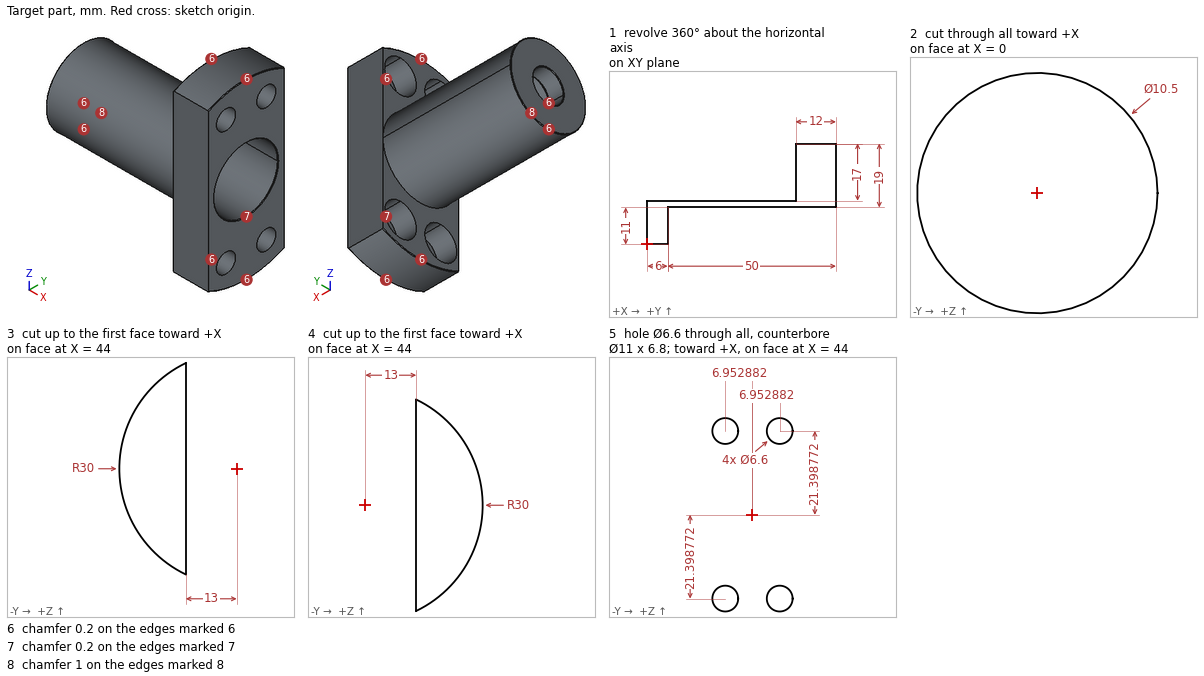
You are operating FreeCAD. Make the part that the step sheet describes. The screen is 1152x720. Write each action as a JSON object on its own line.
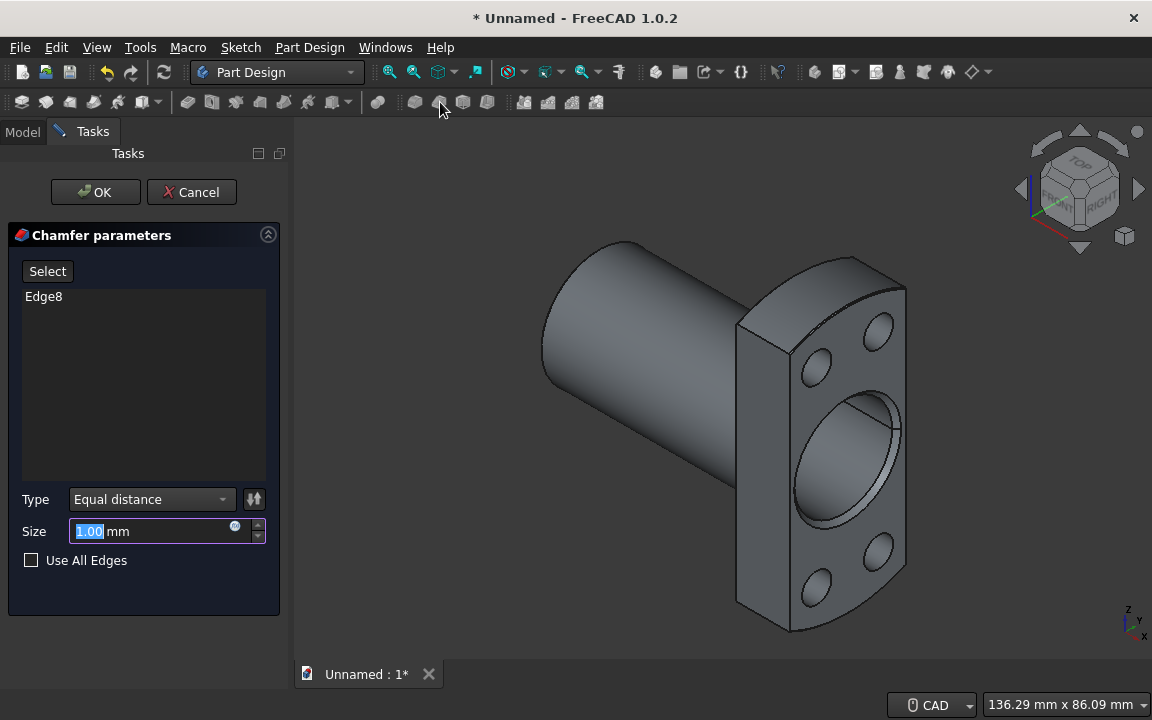
{"action": "type", "text": "0.2"}
{"action": "key", "text": "Tab"}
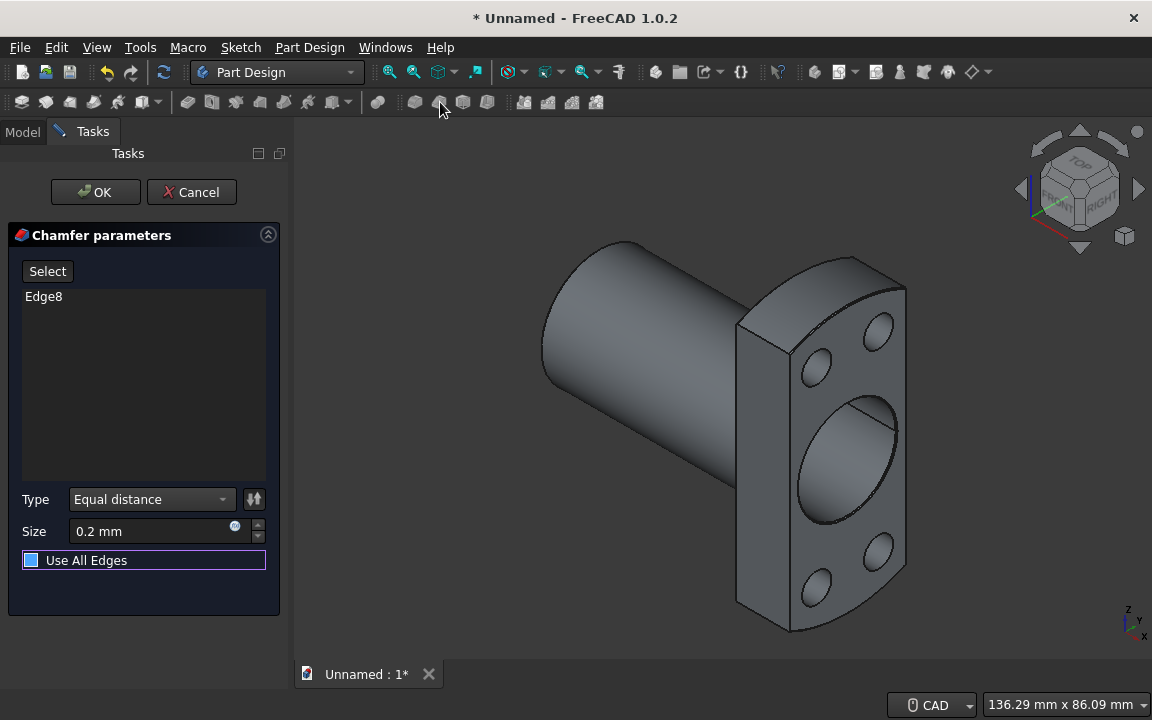
{"action": "left_click", "coordinate": [96, 192]}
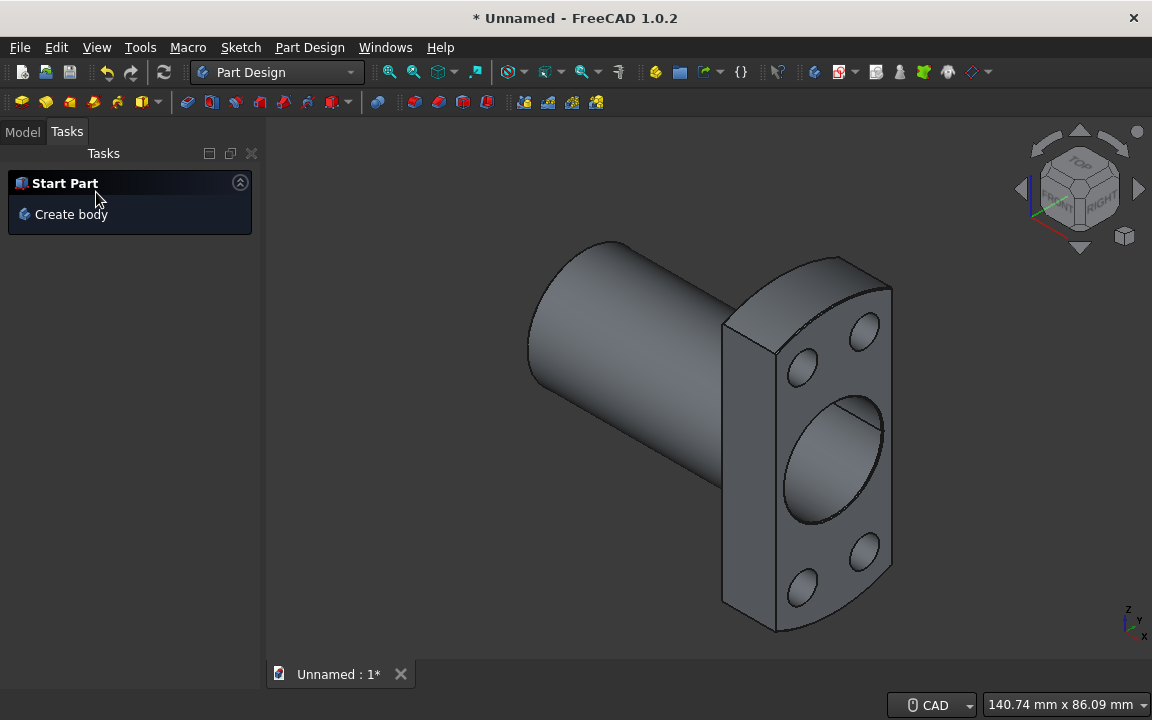
{"action": "key", "text": "2"}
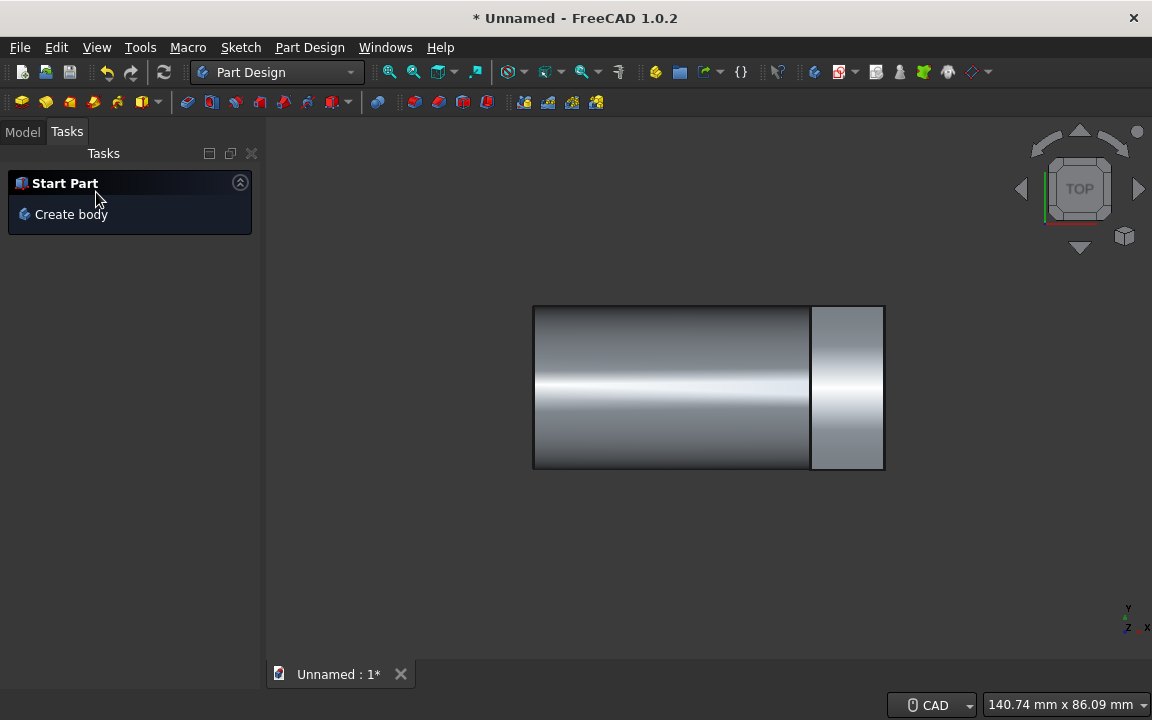
{"action": "left_click", "coordinate": [390, 72]}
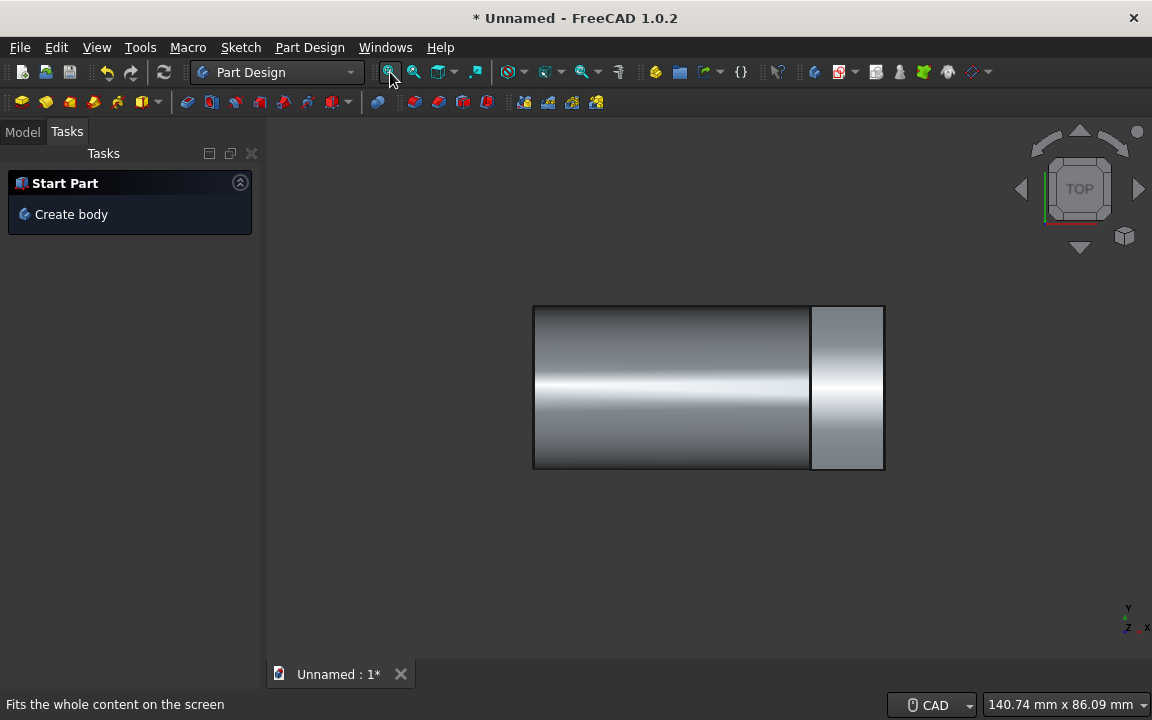
{"action": "key", "text": "0"}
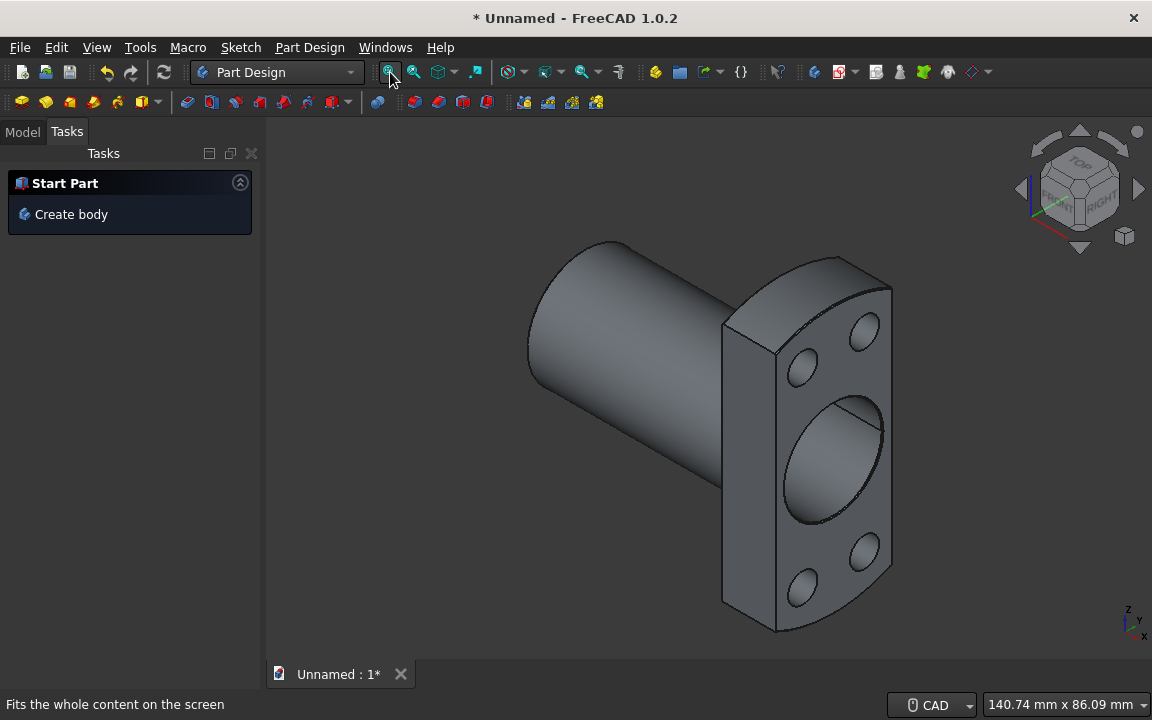
{"action": "key", "text": "1"}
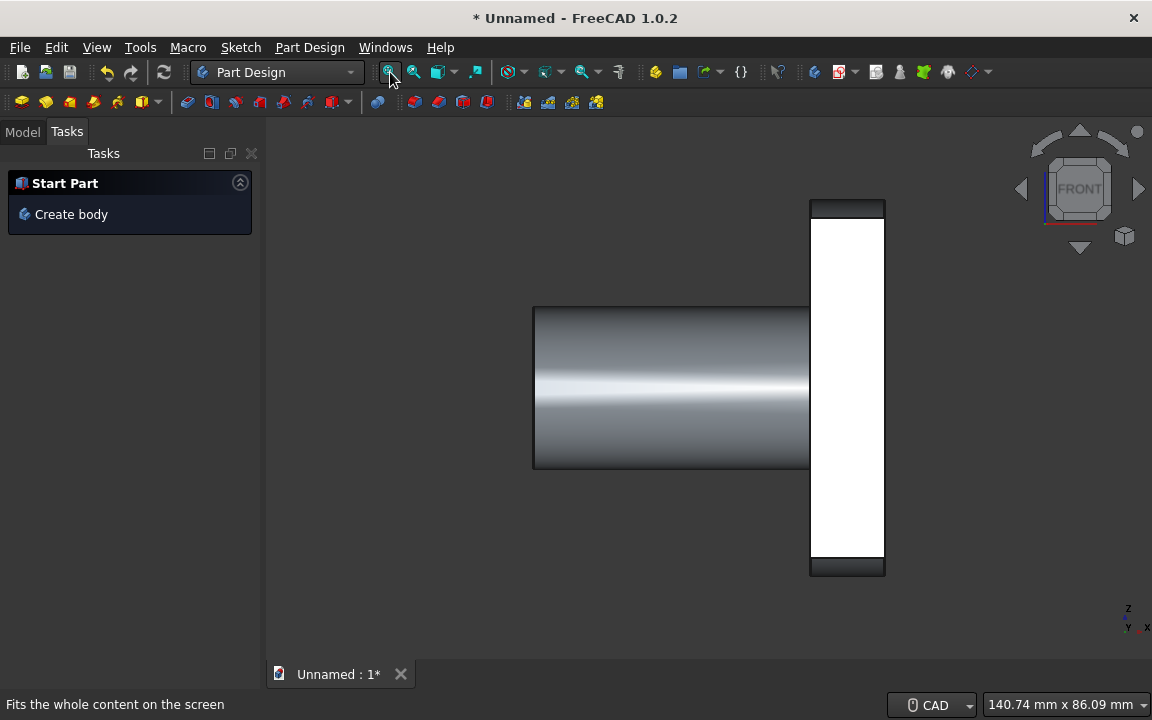
{"action": "key", "text": "3"}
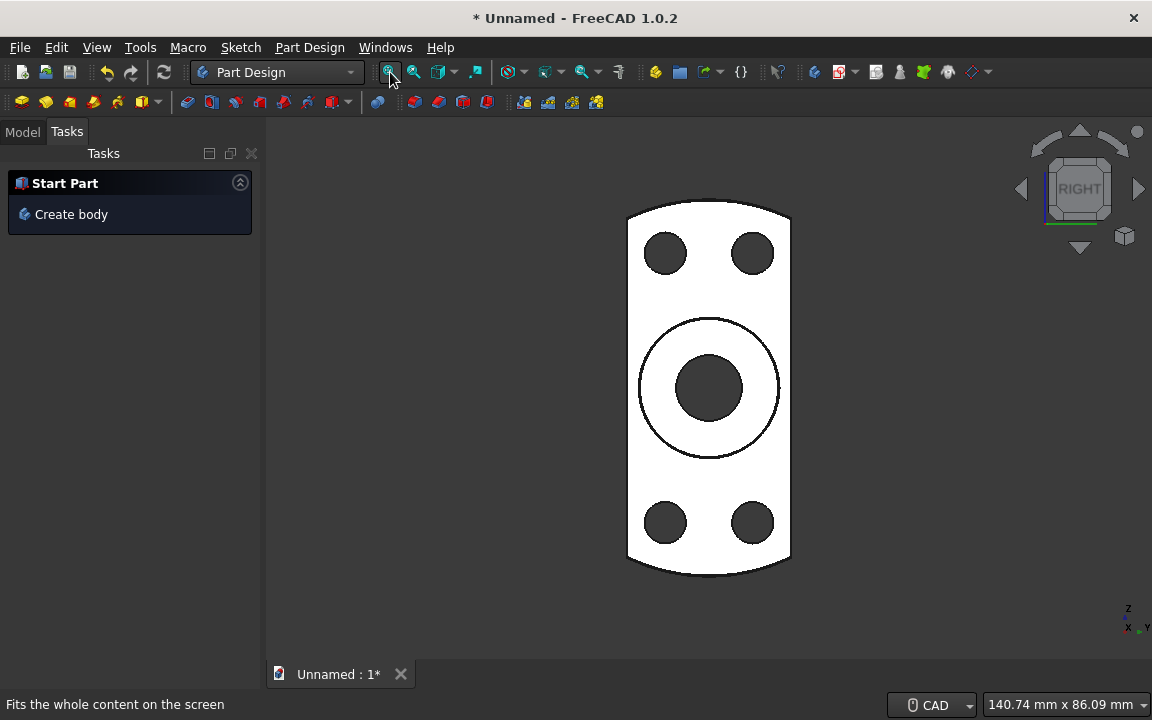
{"action": "left_click", "coordinate": [742, 387]}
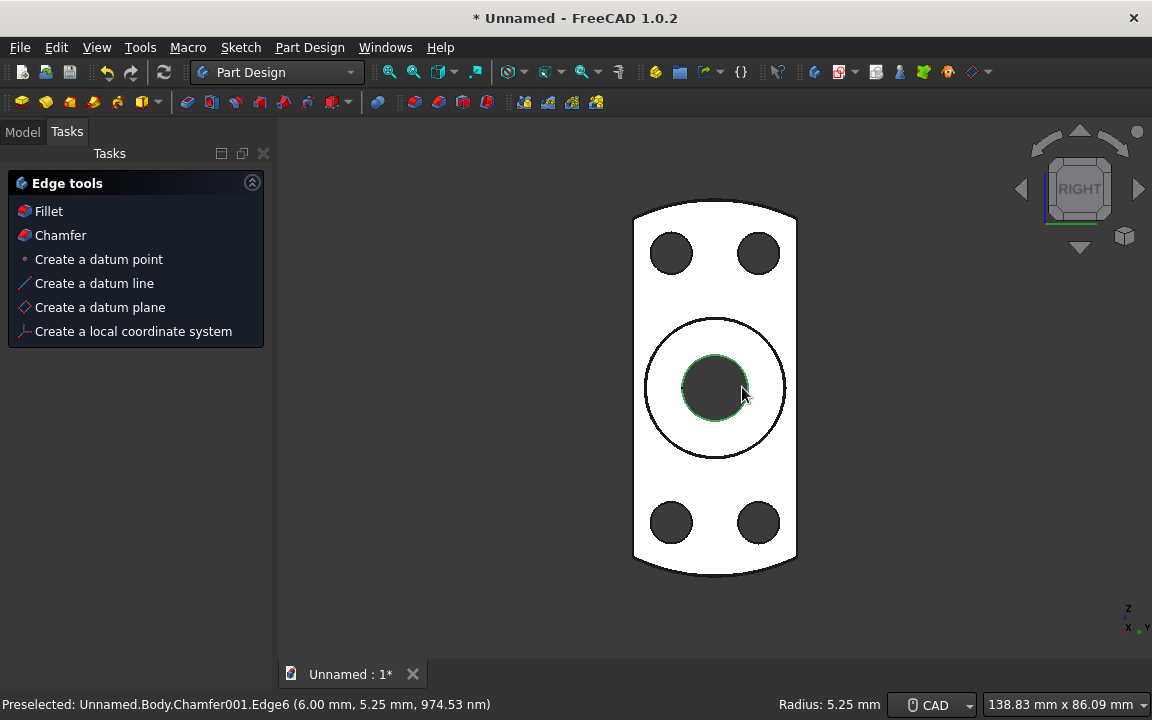
{"action": "left_click", "coordinate": [440, 102]}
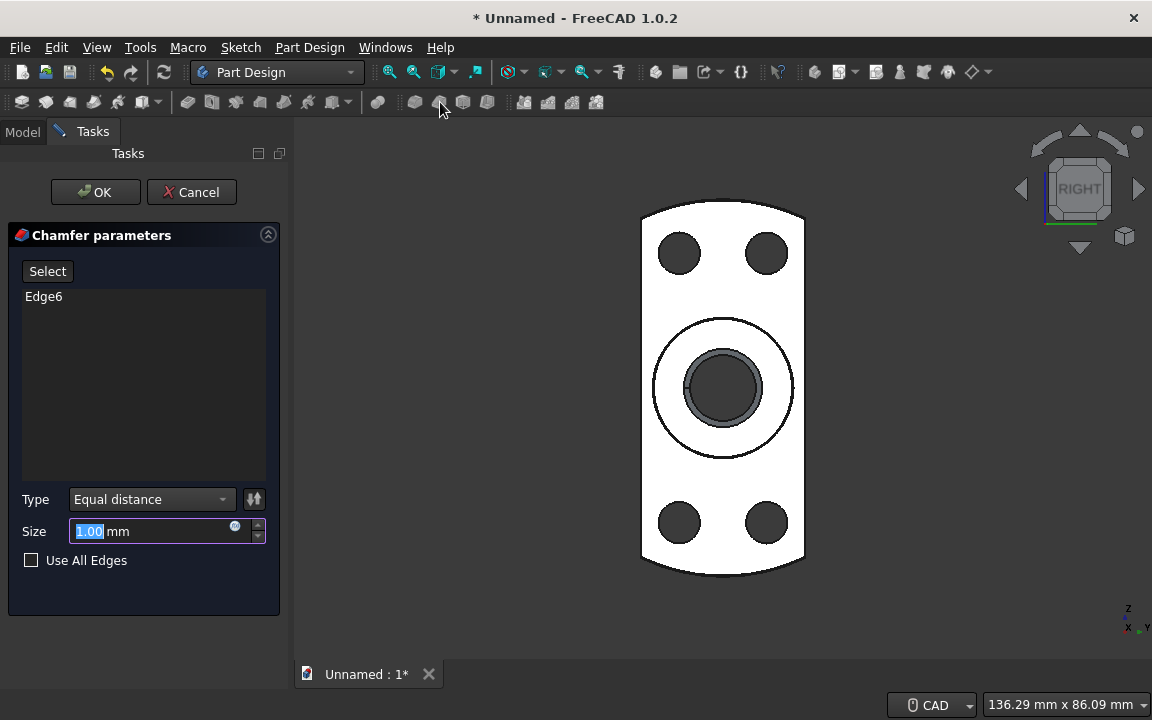
{"action": "type", "text": "1"}
{"action": "key", "text": "Tab"}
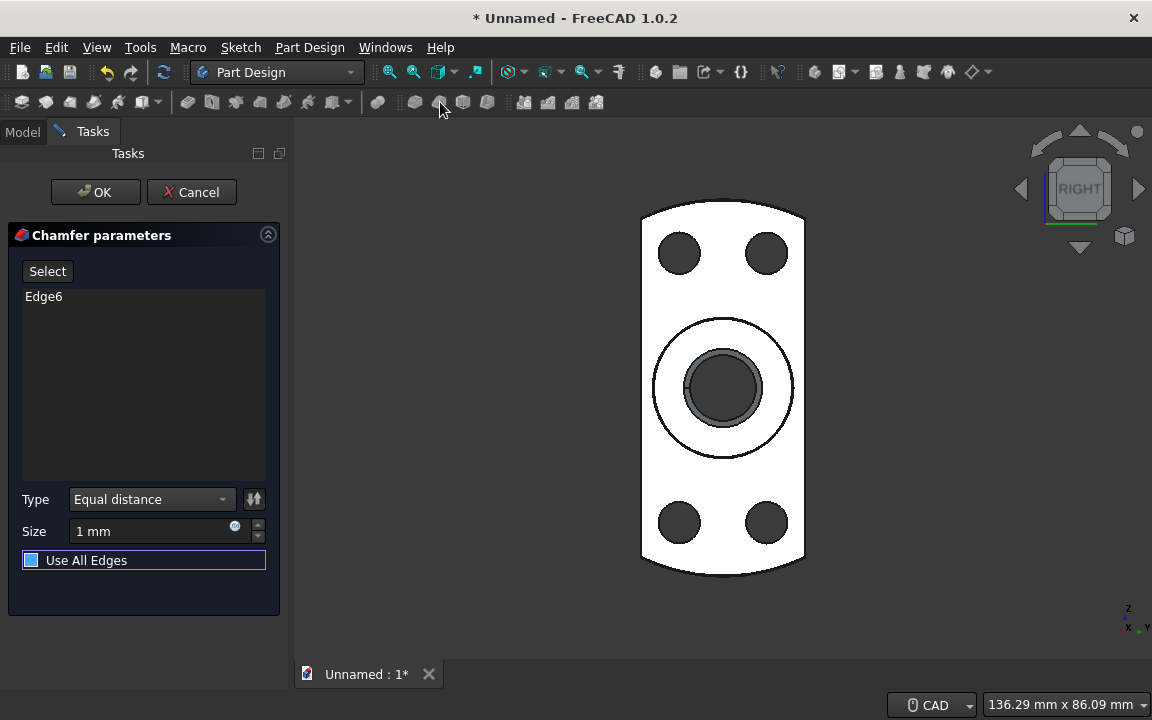
{"action": "left_click", "coordinate": [96, 192]}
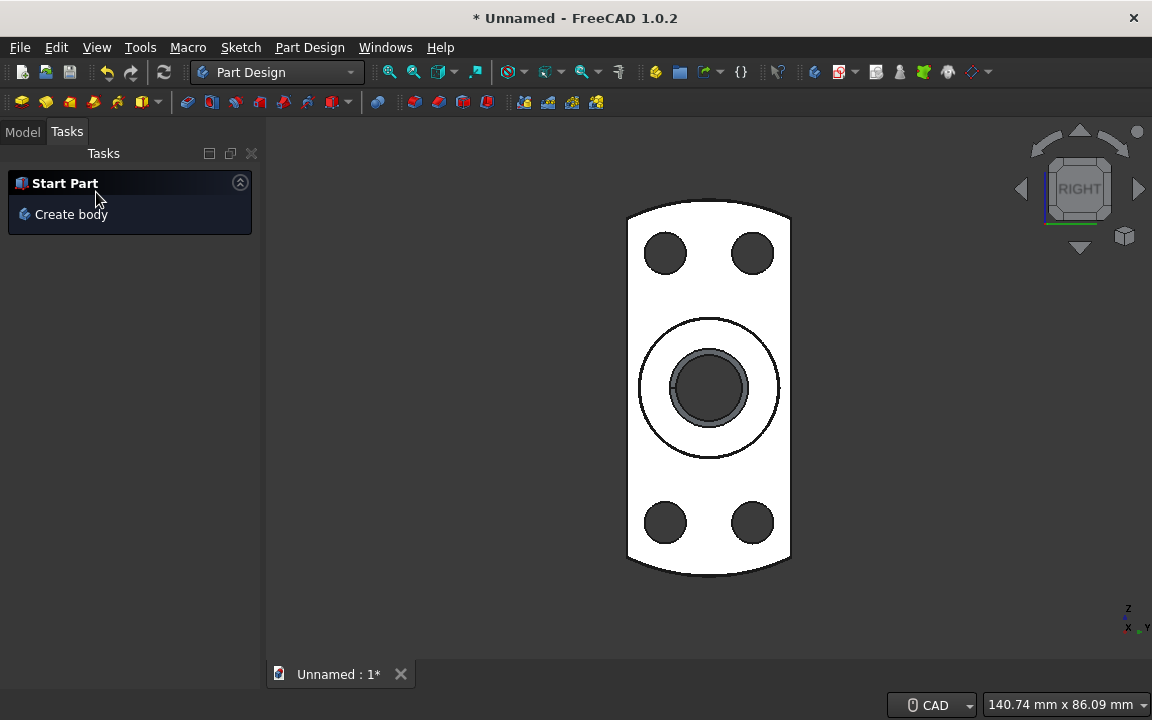
{"action": "key", "text": "0"}